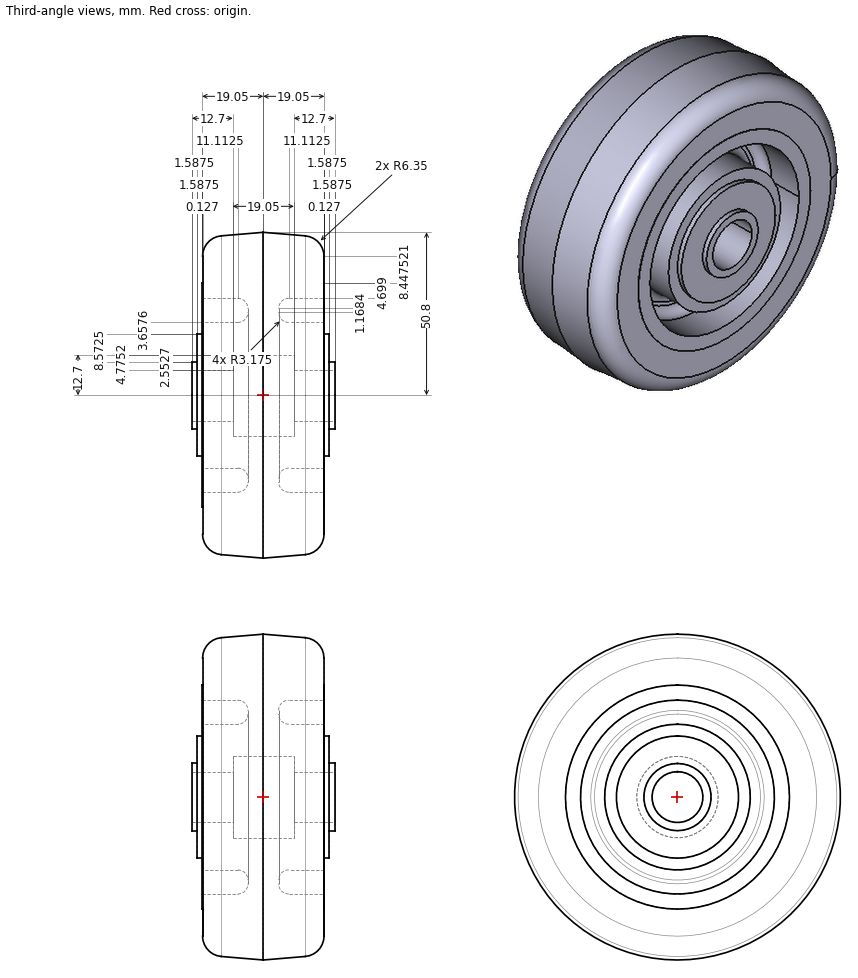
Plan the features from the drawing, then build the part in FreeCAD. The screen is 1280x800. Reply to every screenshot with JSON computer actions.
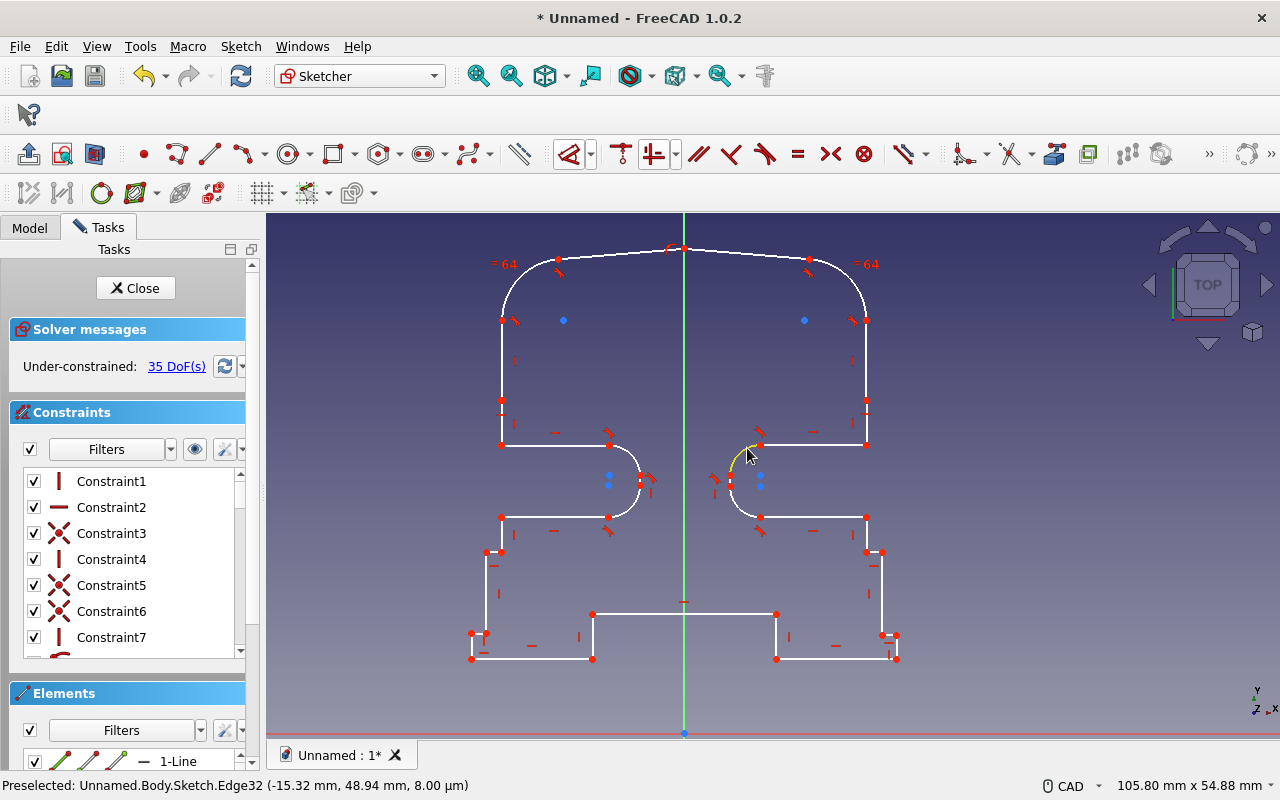
{"action": "left_click", "coordinate": [747, 448]}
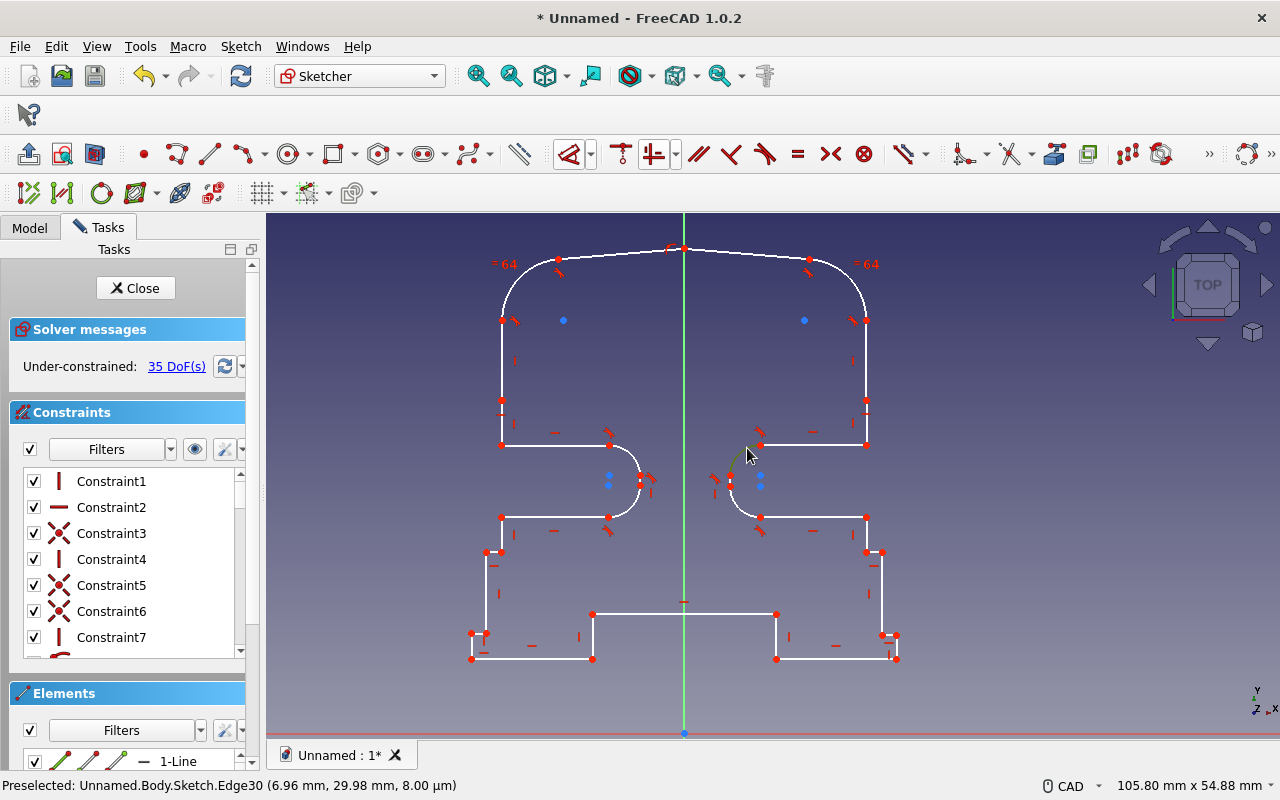
{"action": "left_click", "coordinate": [637, 462]}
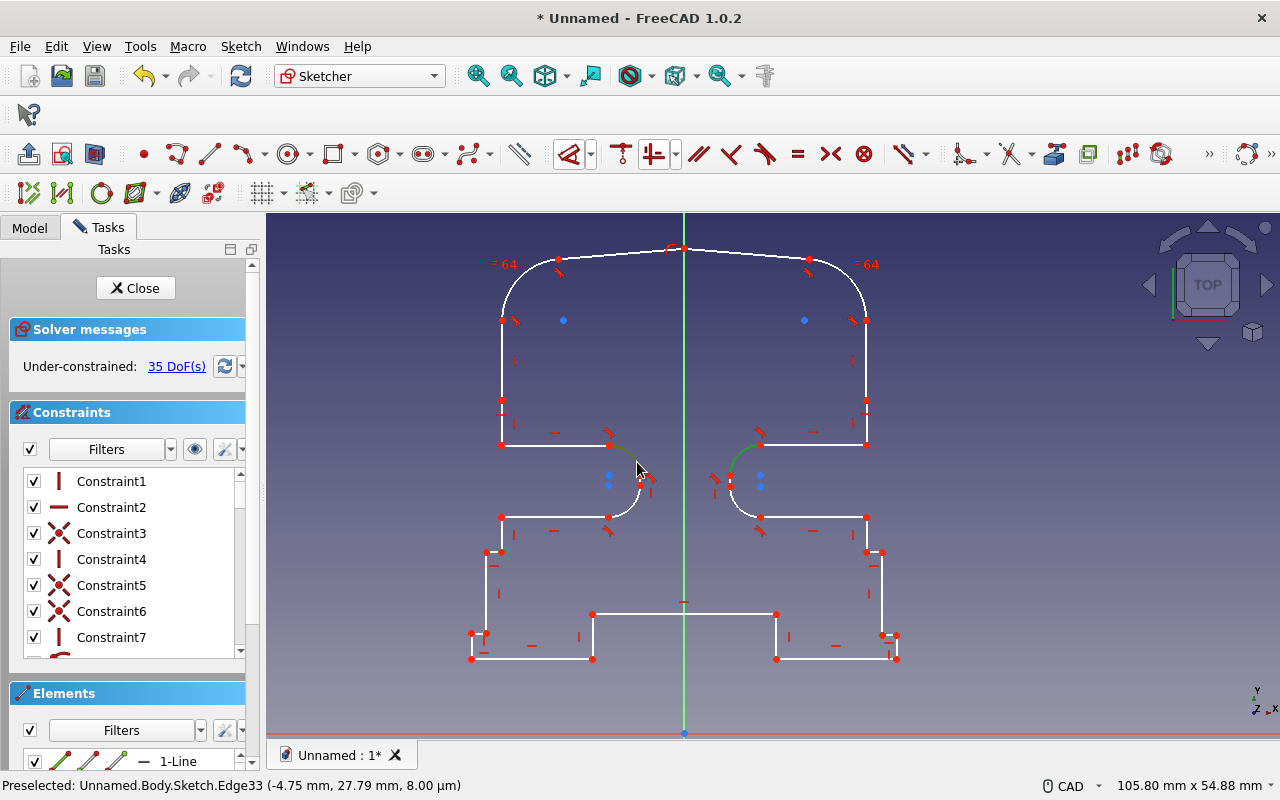
{"action": "left_click", "coordinate": [623, 514]}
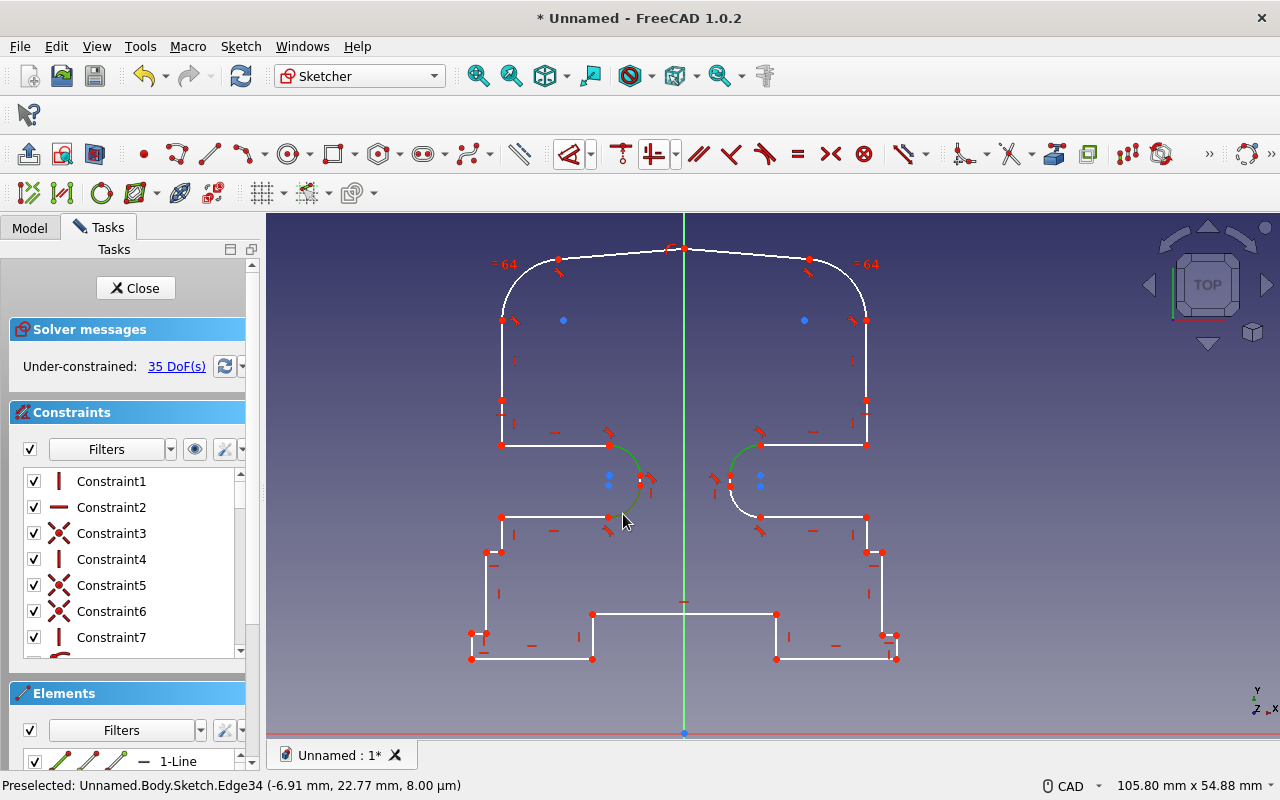
{"action": "left_click", "coordinate": [734, 501]}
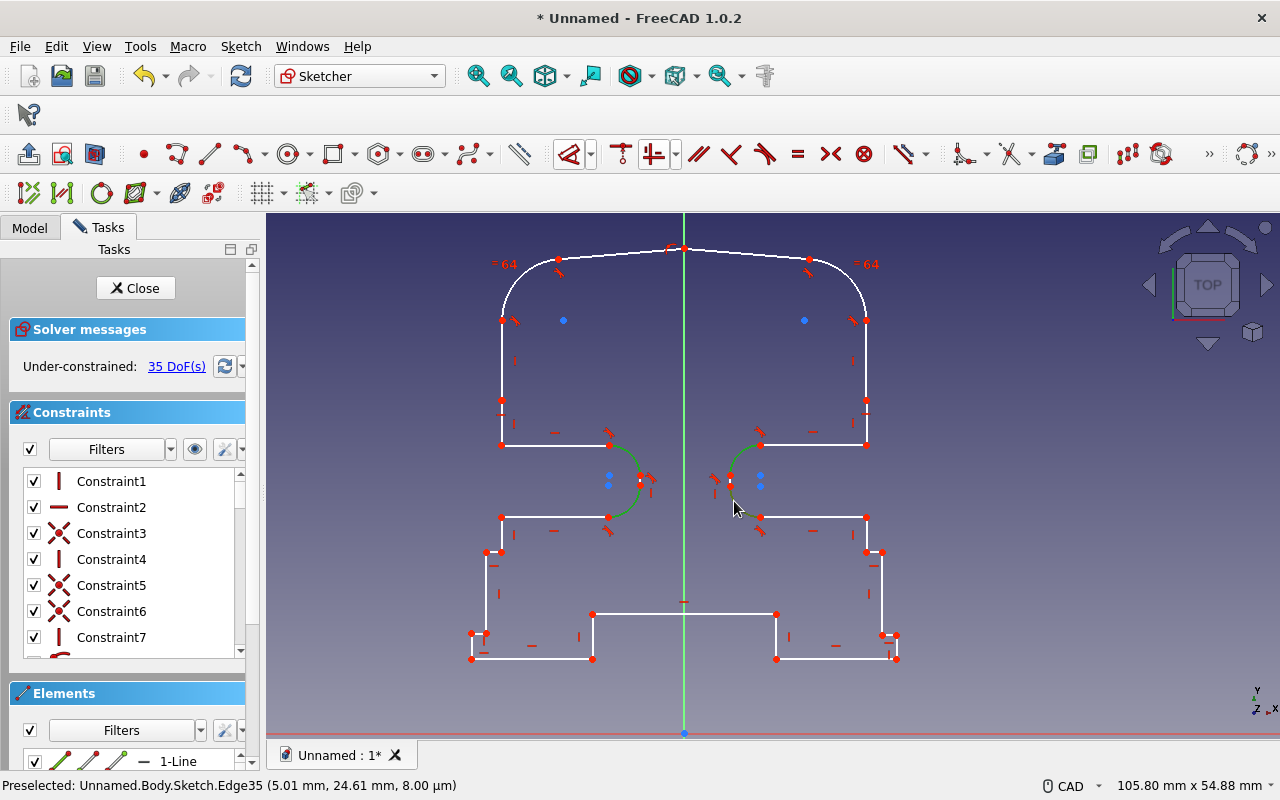
{"action": "left_click", "coordinate": [798, 154]}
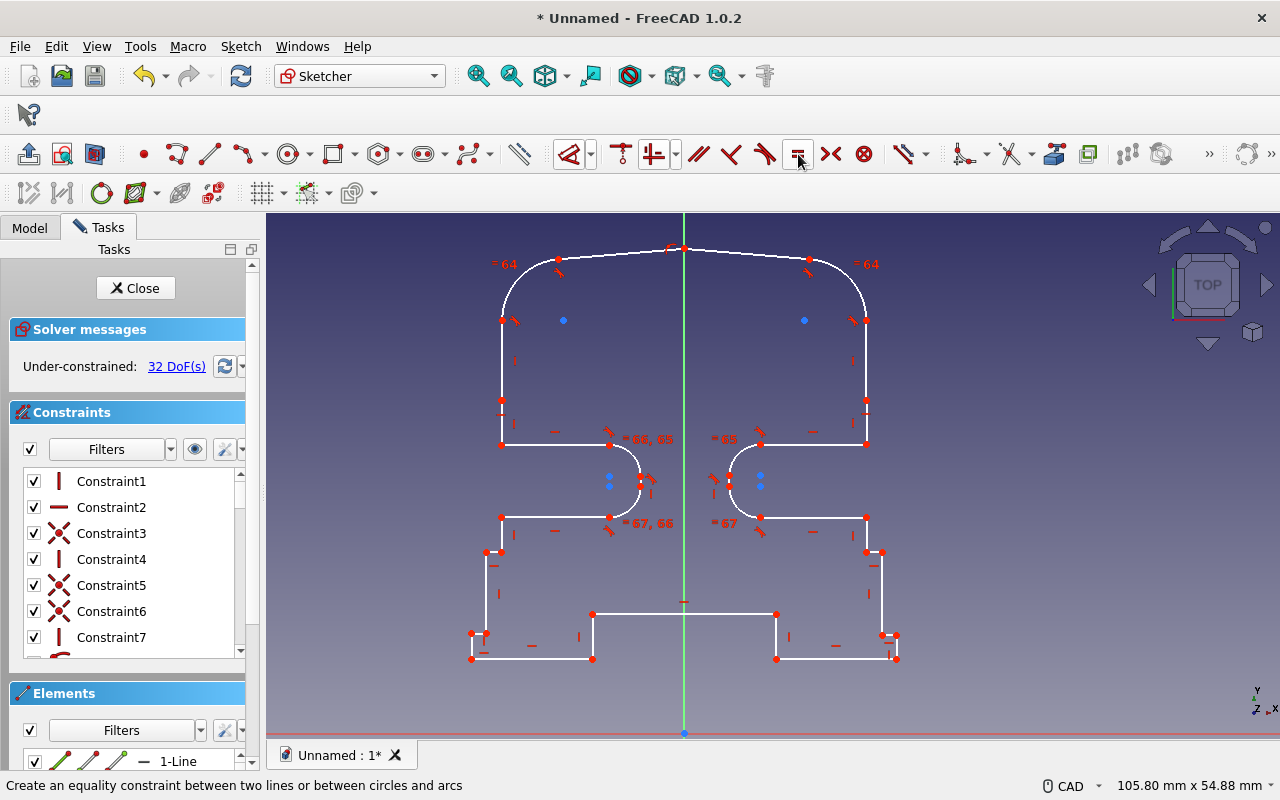
{"action": "scroll", "coordinate": [746, 448], "scroll_direction": "up", "scroll_amount": 2}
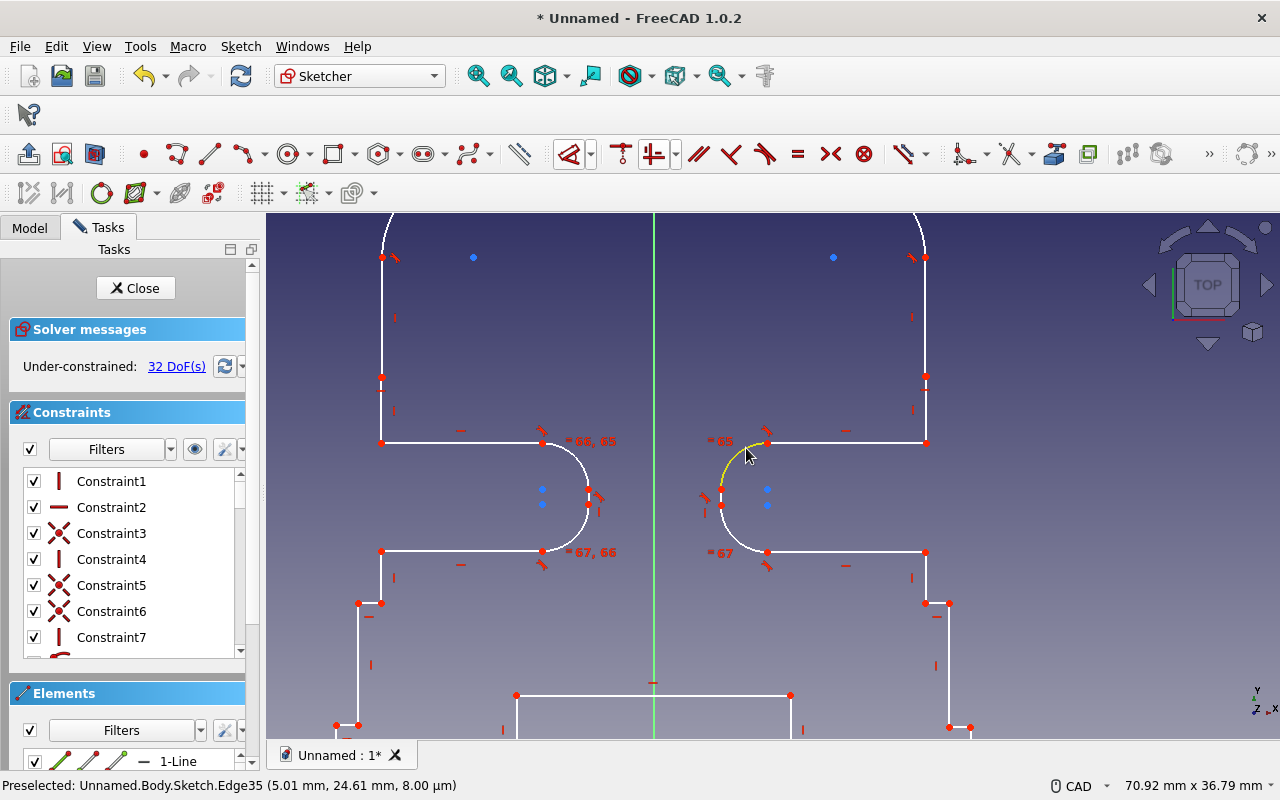
{"action": "left_click", "coordinate": [746, 448]}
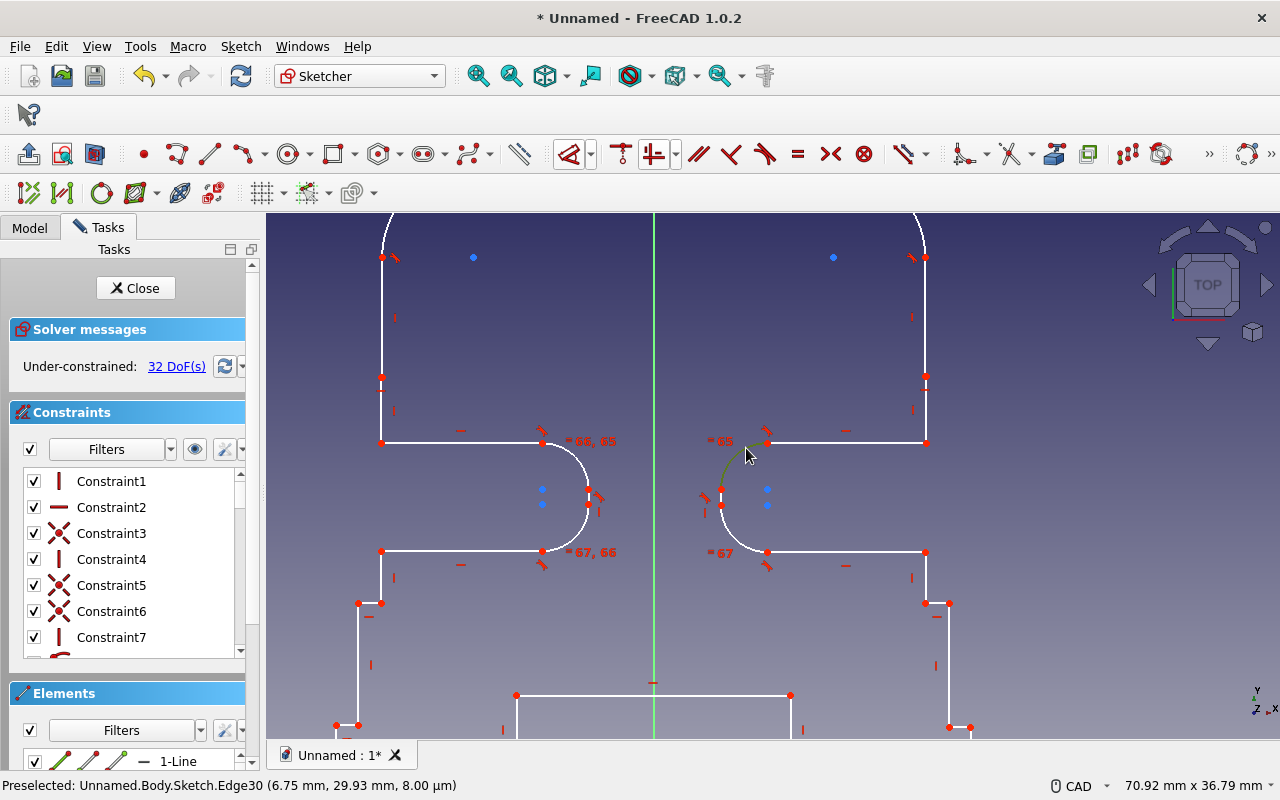
{"action": "key", "text": "k r"}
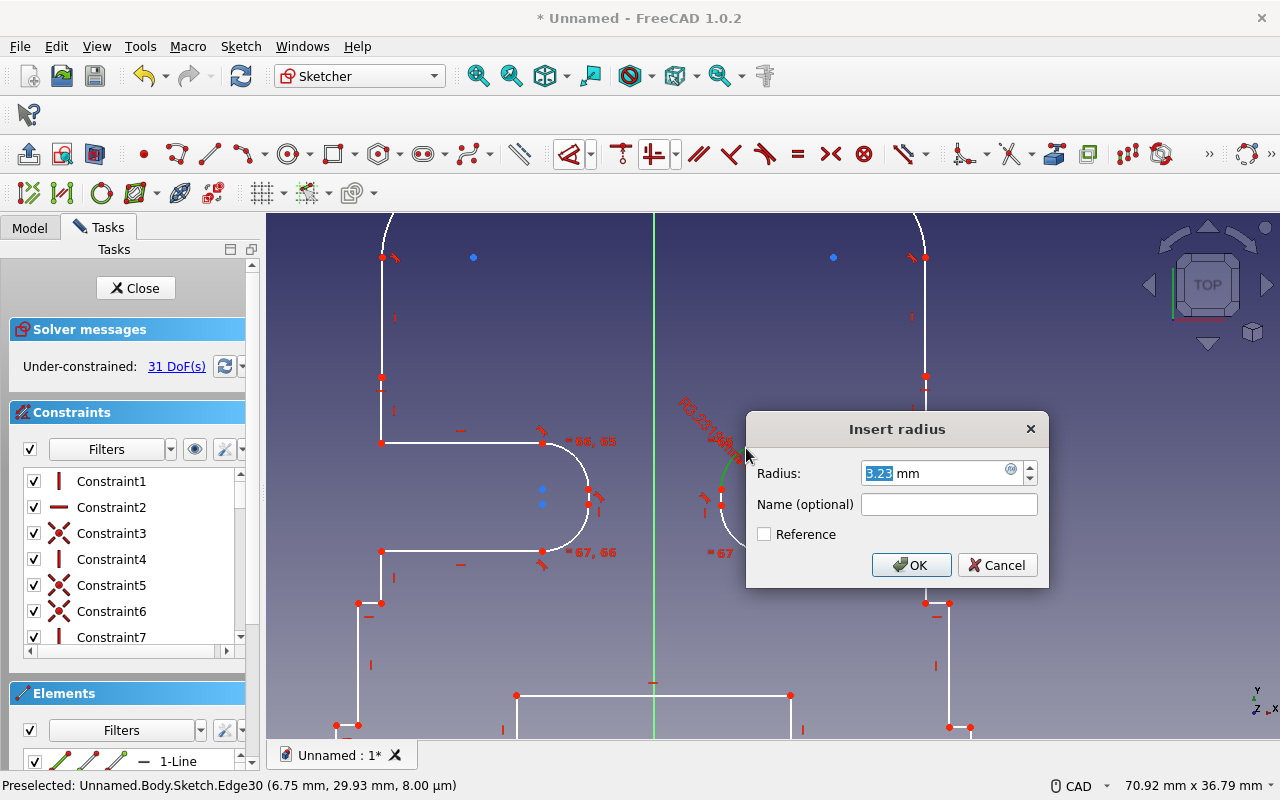
{"action": "type", "text": "3.175"}
{"action": "key", "text": "Return"}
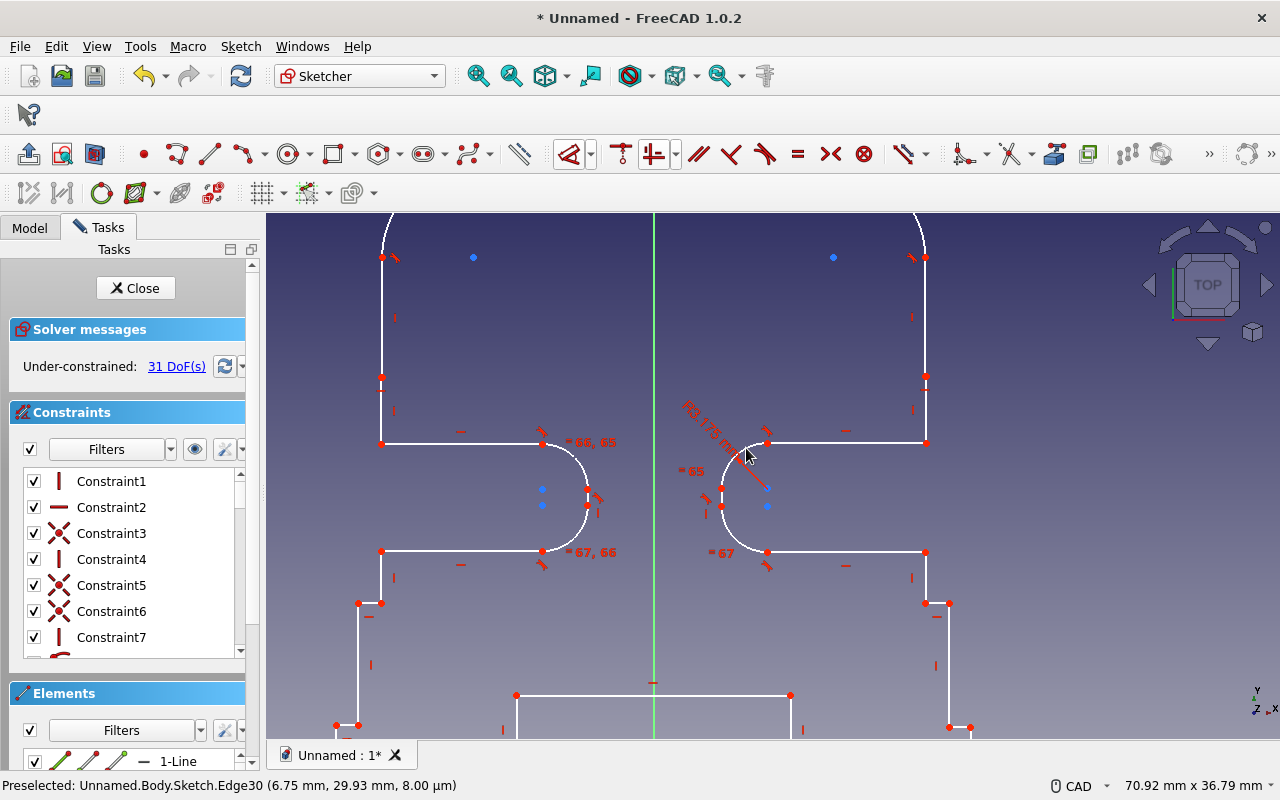
{"action": "scroll", "coordinate": [746, 447], "scroll_direction": "down", "scroll_amount": 4}